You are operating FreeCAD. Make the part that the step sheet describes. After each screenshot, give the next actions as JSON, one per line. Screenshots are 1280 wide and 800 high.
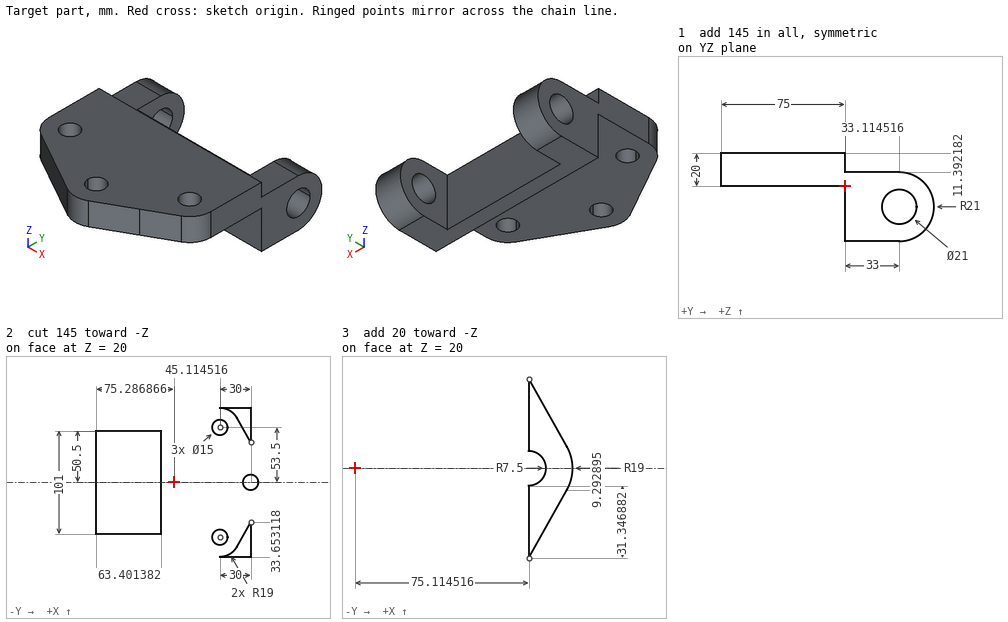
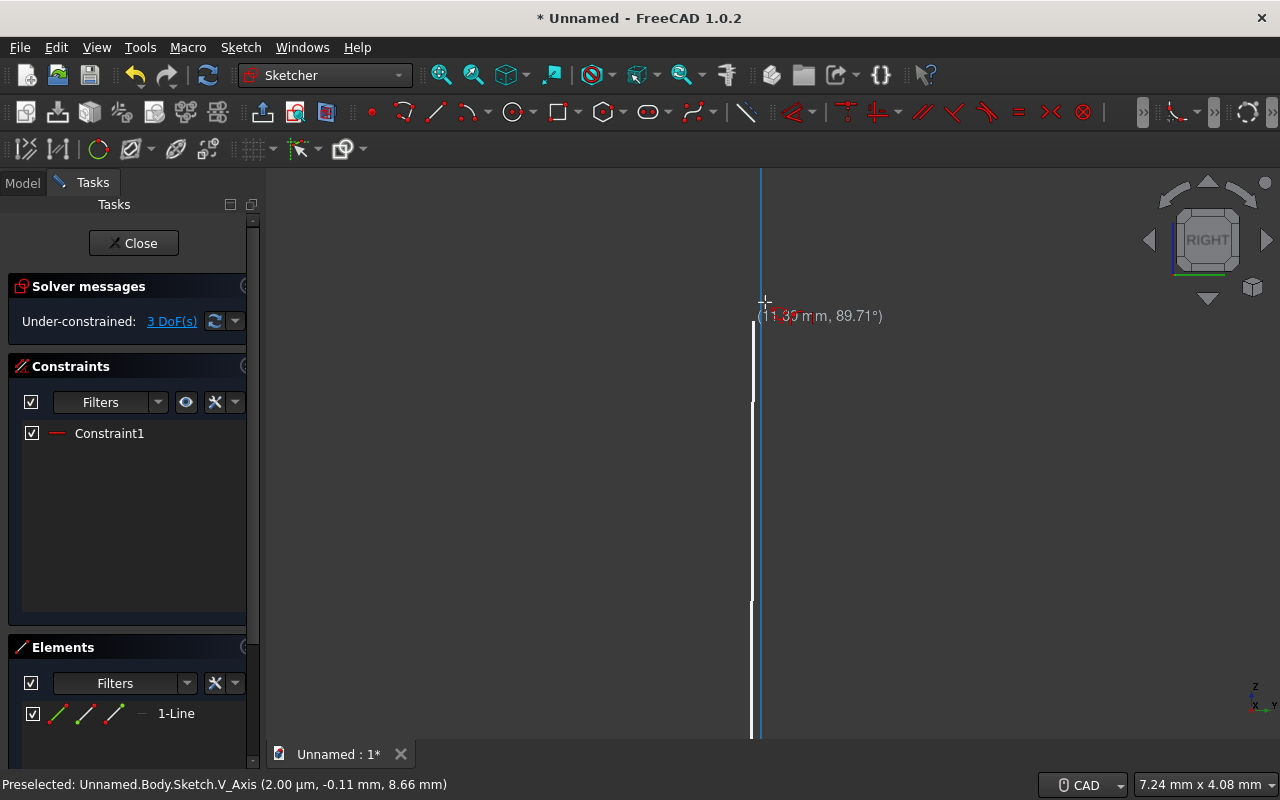
{"action": "left_click", "coordinate": [745, 292]}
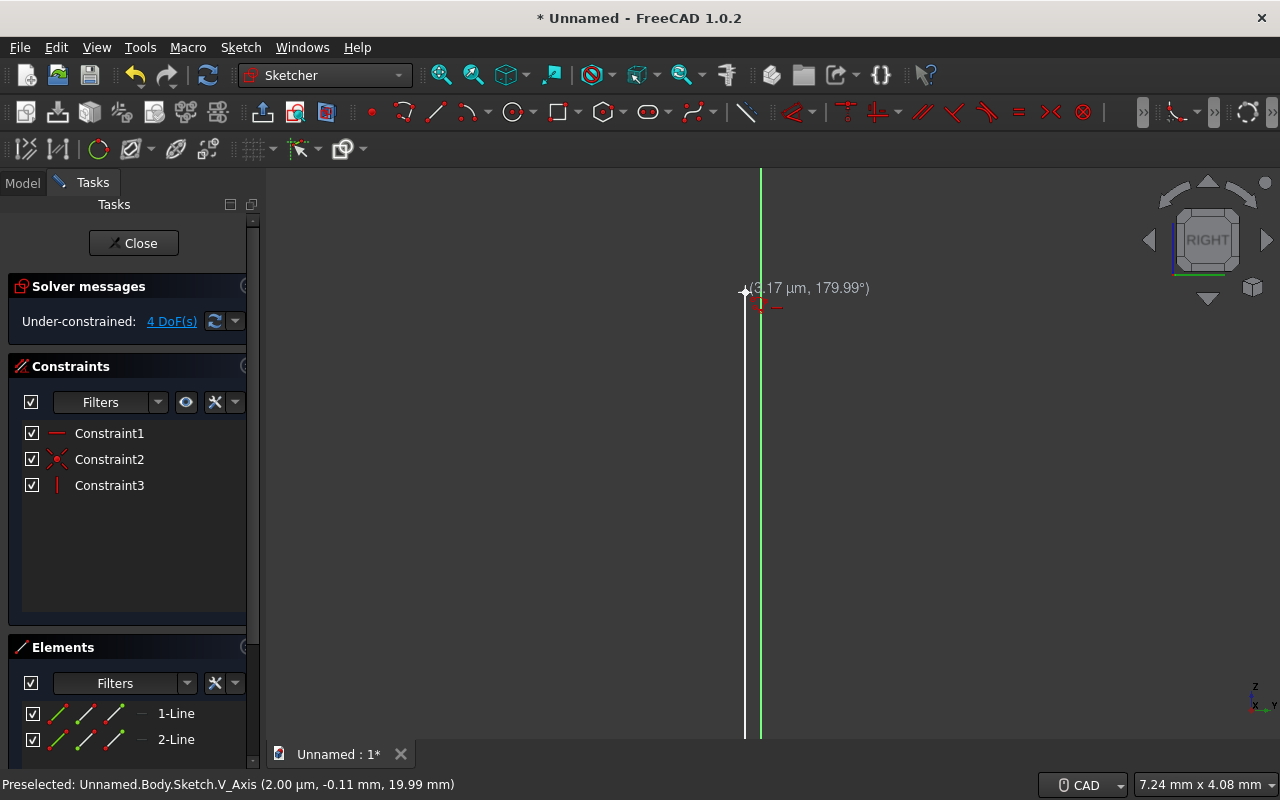
{"action": "scroll", "coordinate": [765, 301], "scroll_direction": "down", "scroll_amount": 16}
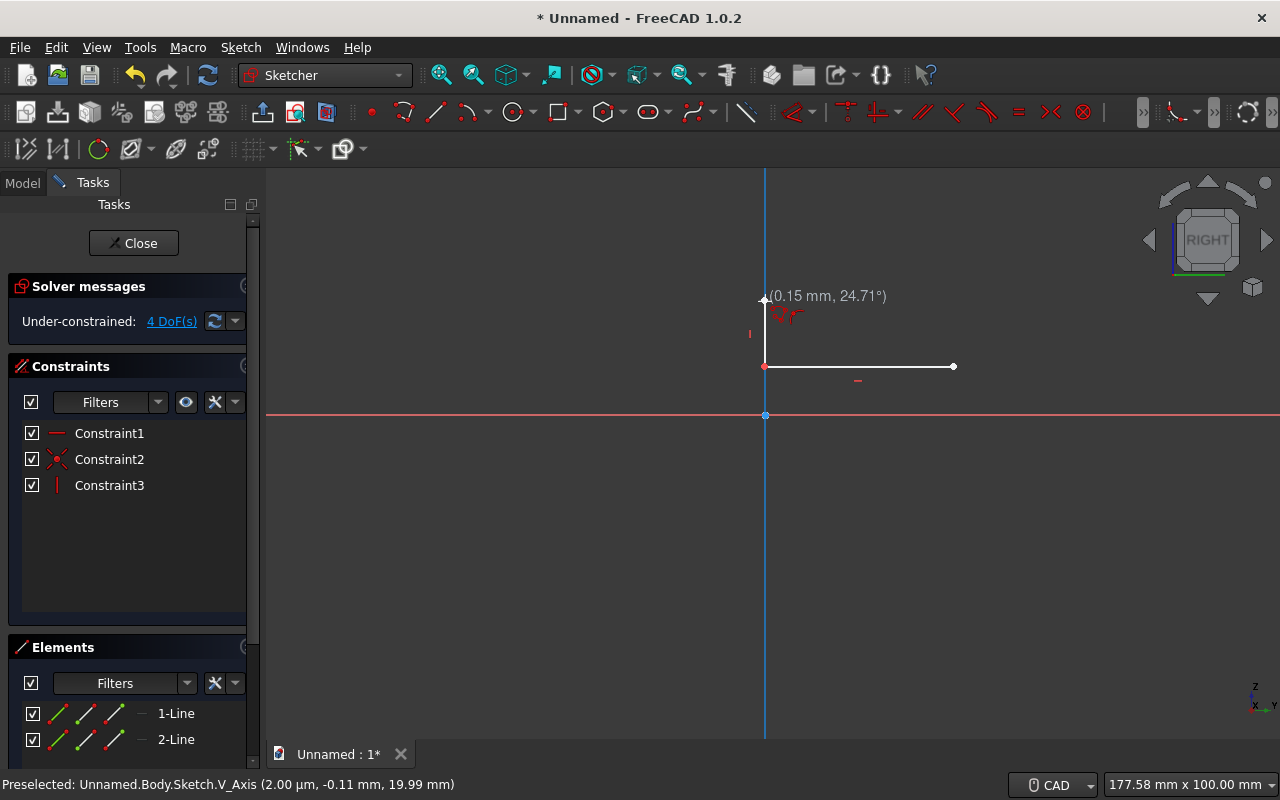
{"action": "left_click", "coordinate": [336, 301]}
{"action": "left_click", "coordinate": [336, 415]}
{"action": "left_click", "coordinate": [765, 415]}
{"action": "left_click", "coordinate": [756, 606]}
{"action": "left_click", "coordinate": [954, 606]}
{"action": "right_click", "coordinate": [954, 606]}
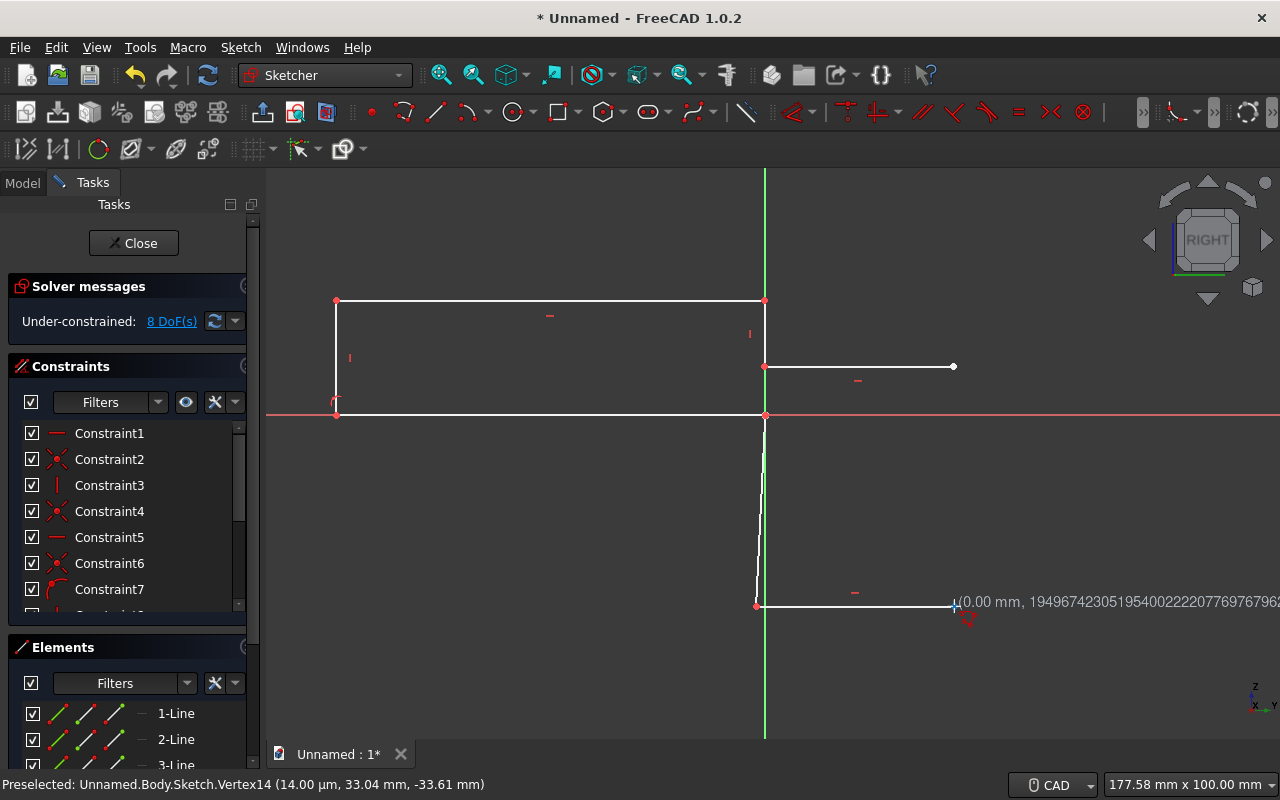
{"action": "left_click", "coordinate": [490, 112]}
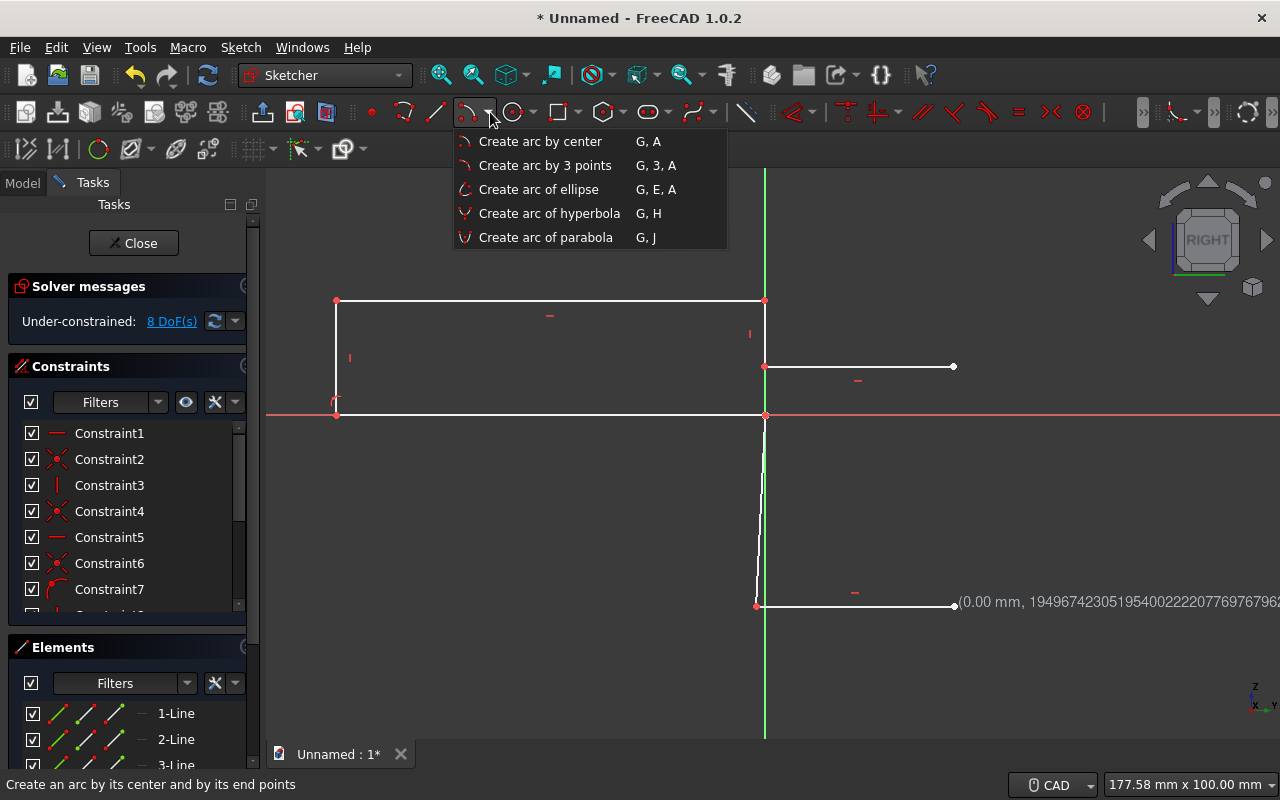
{"action": "left_click", "coordinate": [590, 165]}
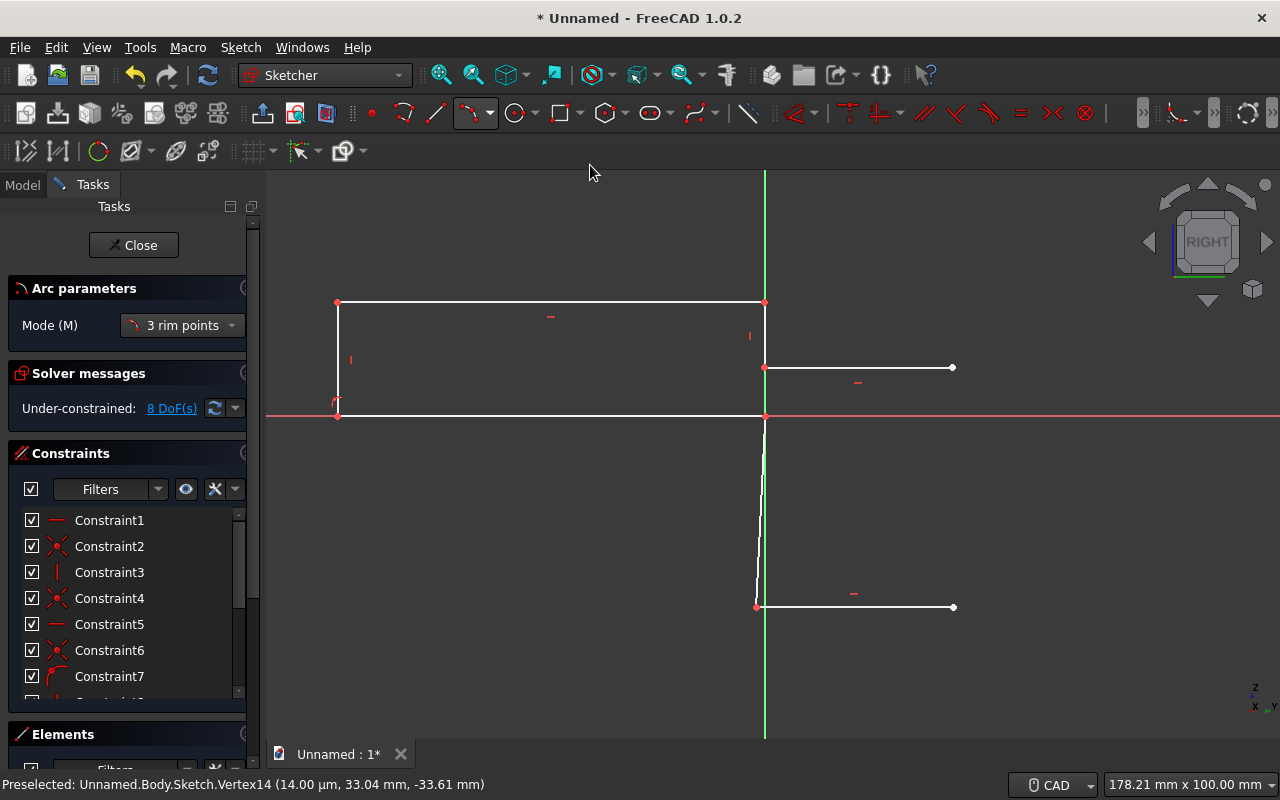
{"action": "left_click", "coordinate": [953, 607]}
{"action": "left_click", "coordinate": [953, 368]}
{"action": "left_click", "coordinate": [1073, 487]}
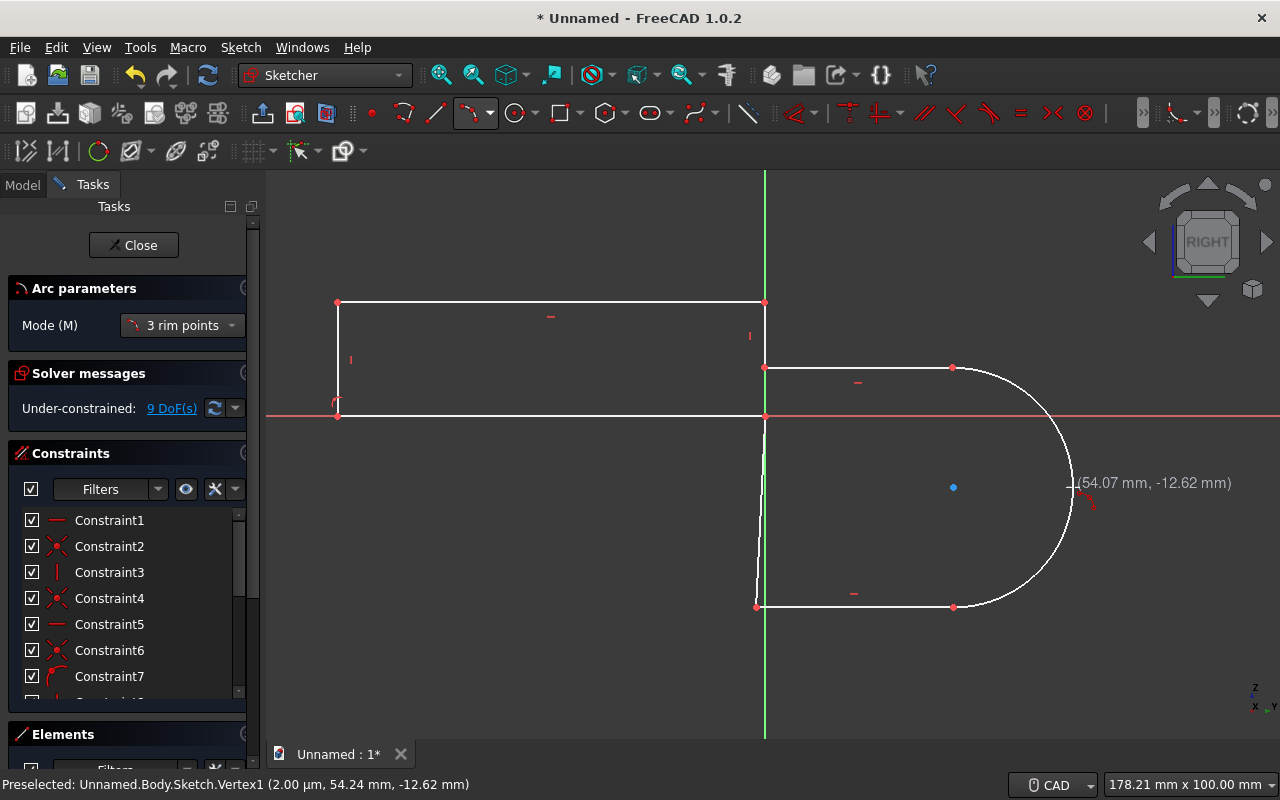
{"action": "left_click", "coordinate": [516, 114]}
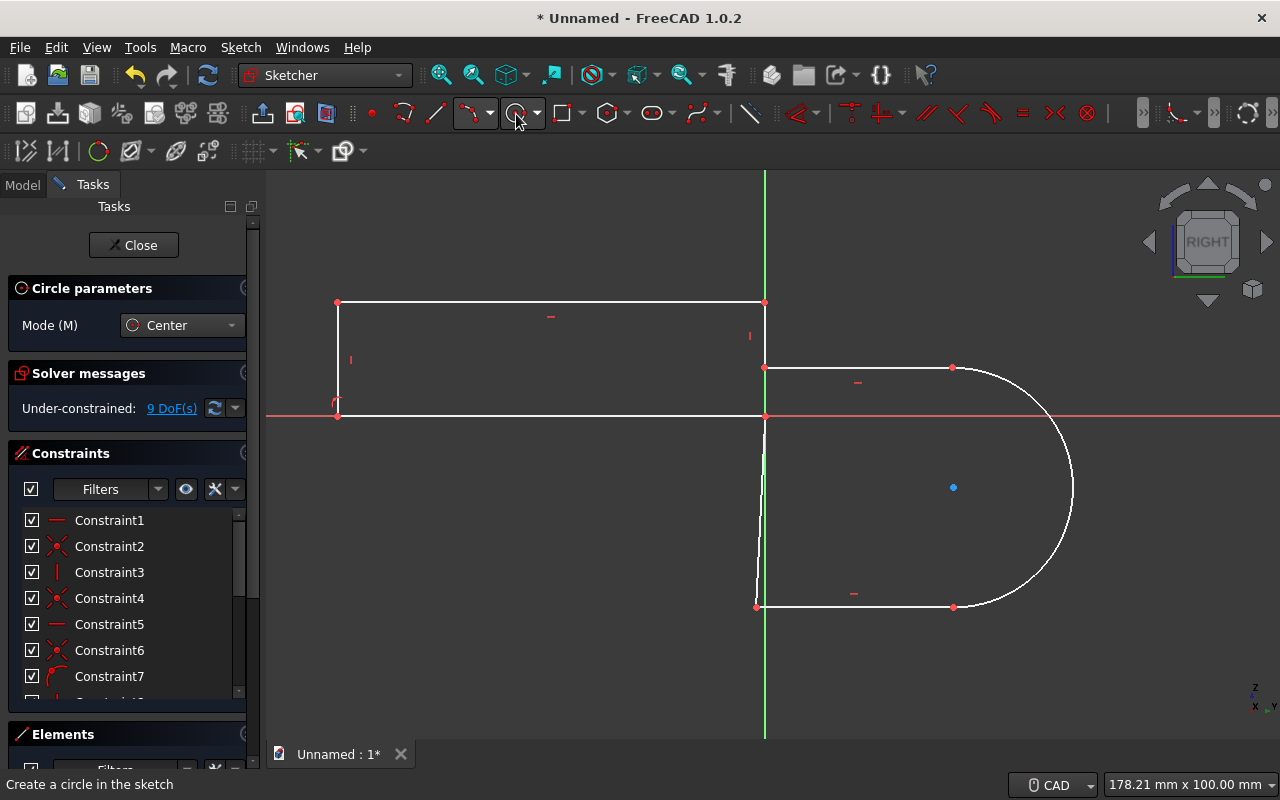
{"action": "left_click", "coordinate": [953, 487]}
{"action": "mouse_move", "coordinate": [995, 444]}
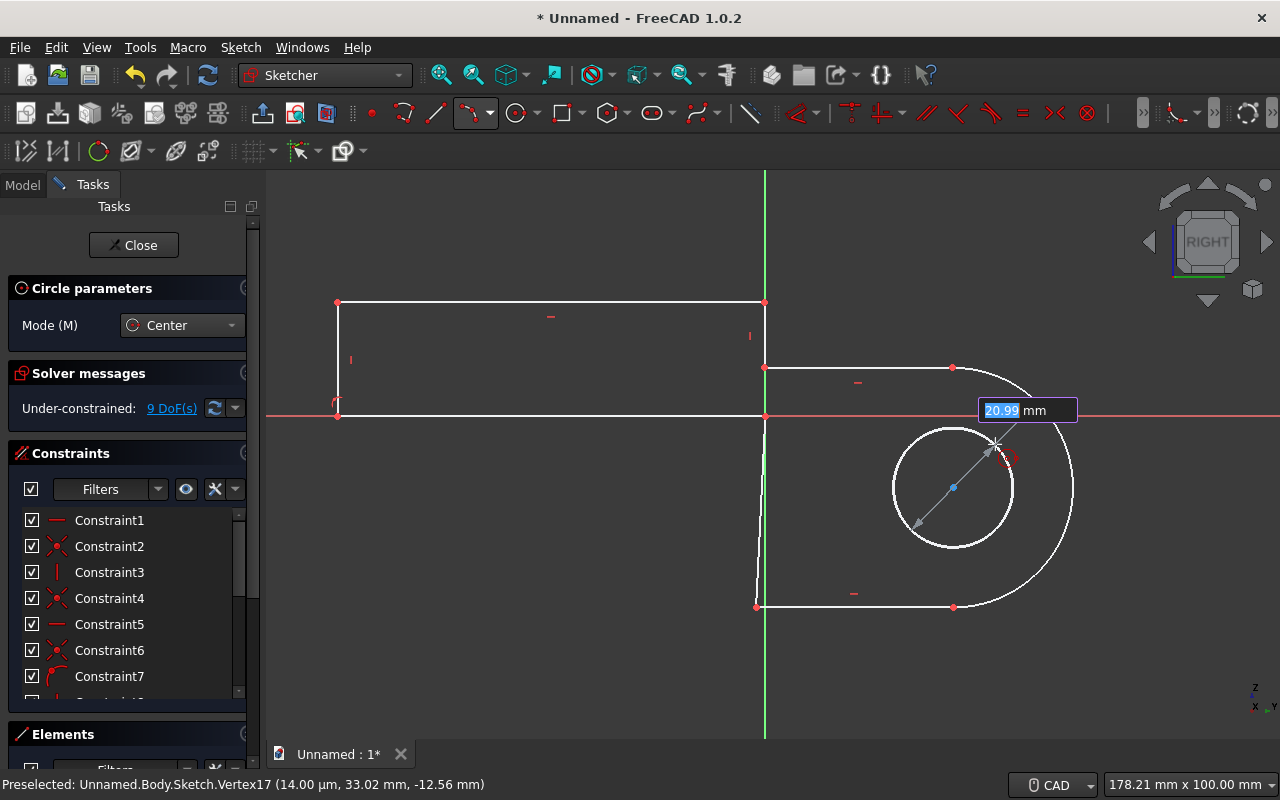
{"action": "type", "text": "21"}
{"action": "key", "text": "Return"}
{"action": "key", "text": "Escape"}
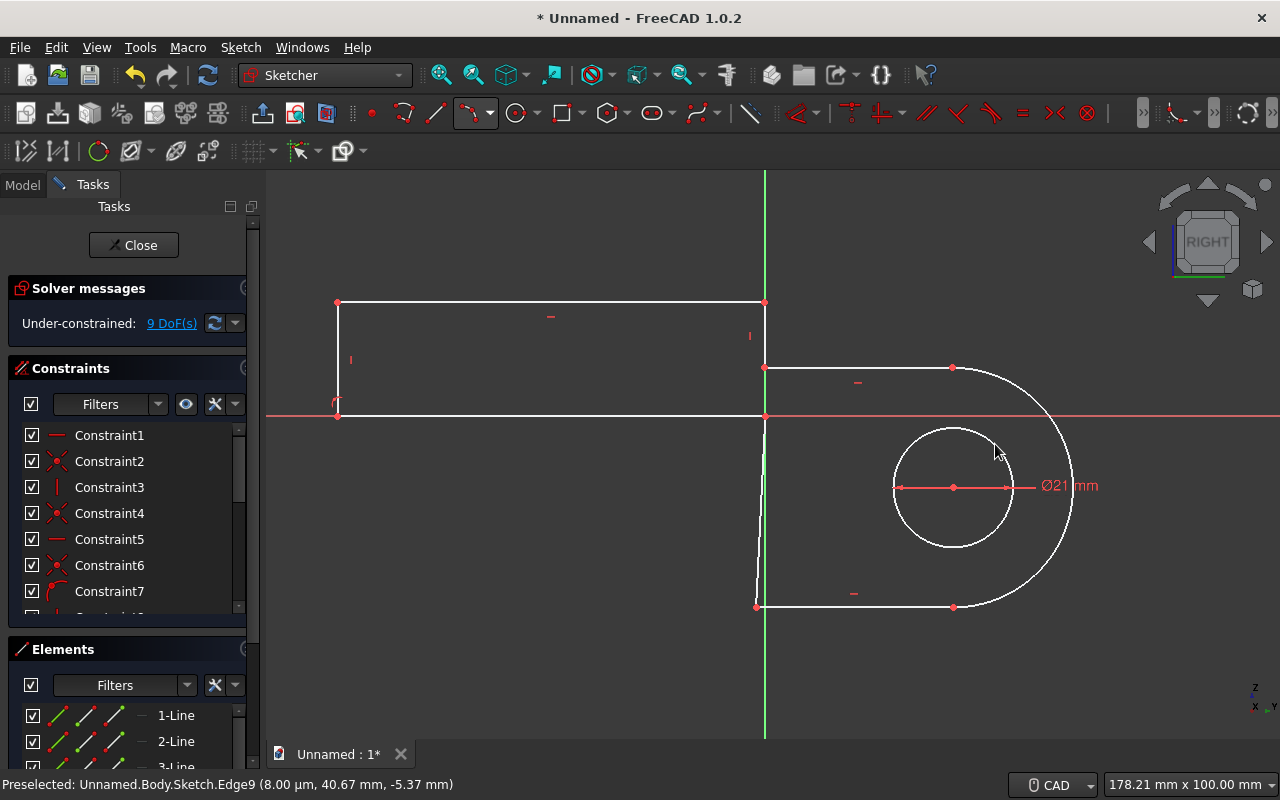
{"action": "left_click", "coordinate": [896, 368]}